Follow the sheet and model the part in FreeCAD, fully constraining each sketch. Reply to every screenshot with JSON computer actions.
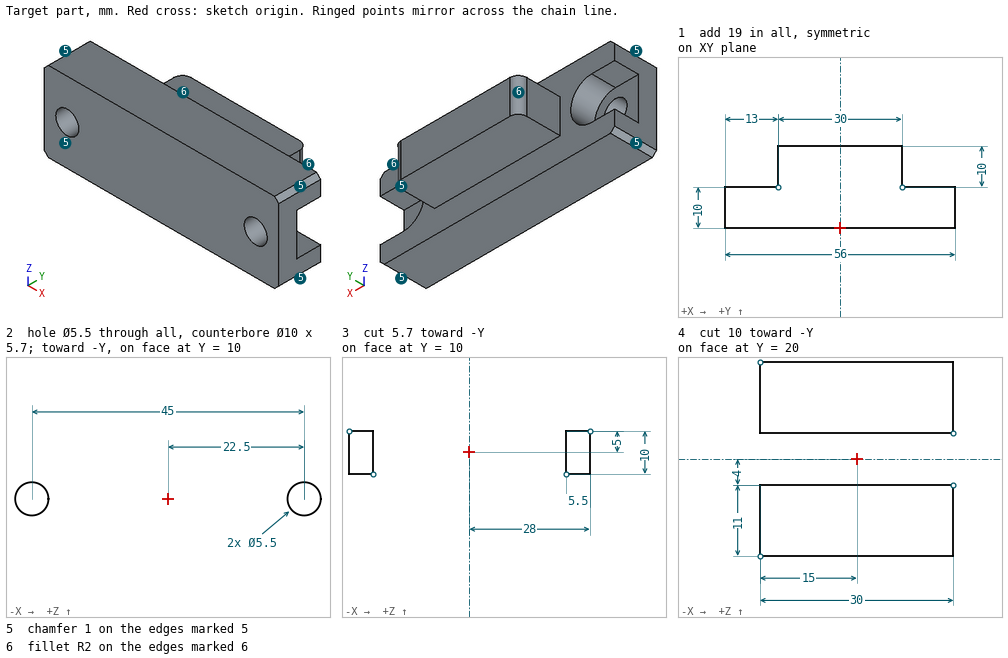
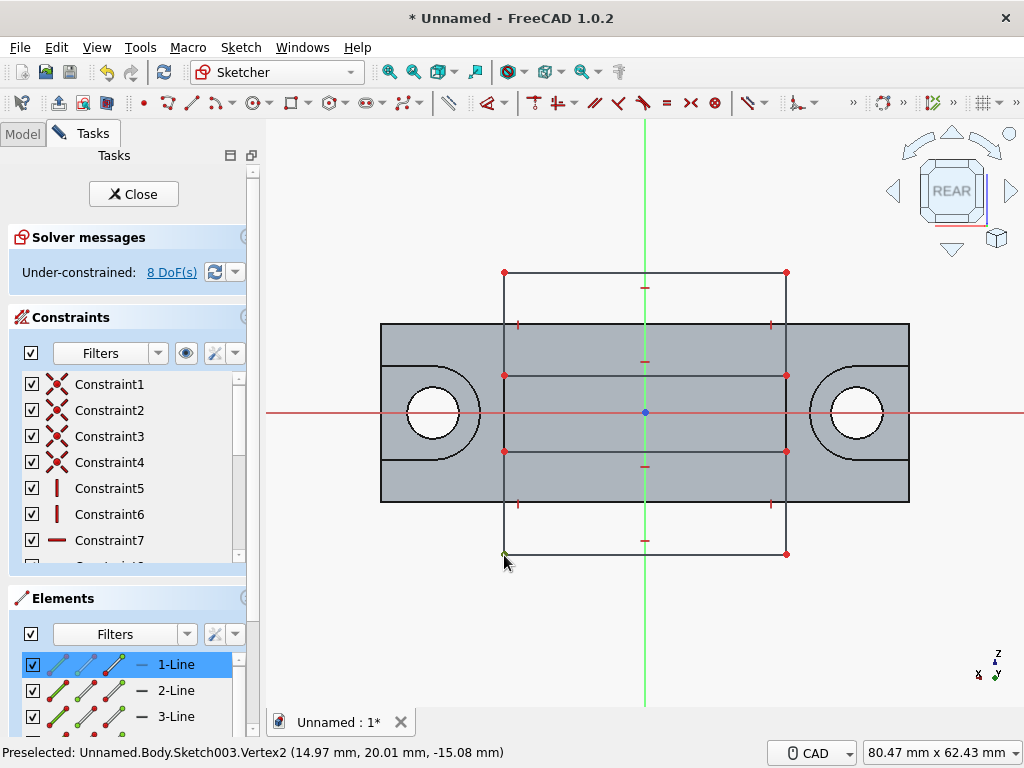
{"action": "left_click", "coordinate": [504, 273]}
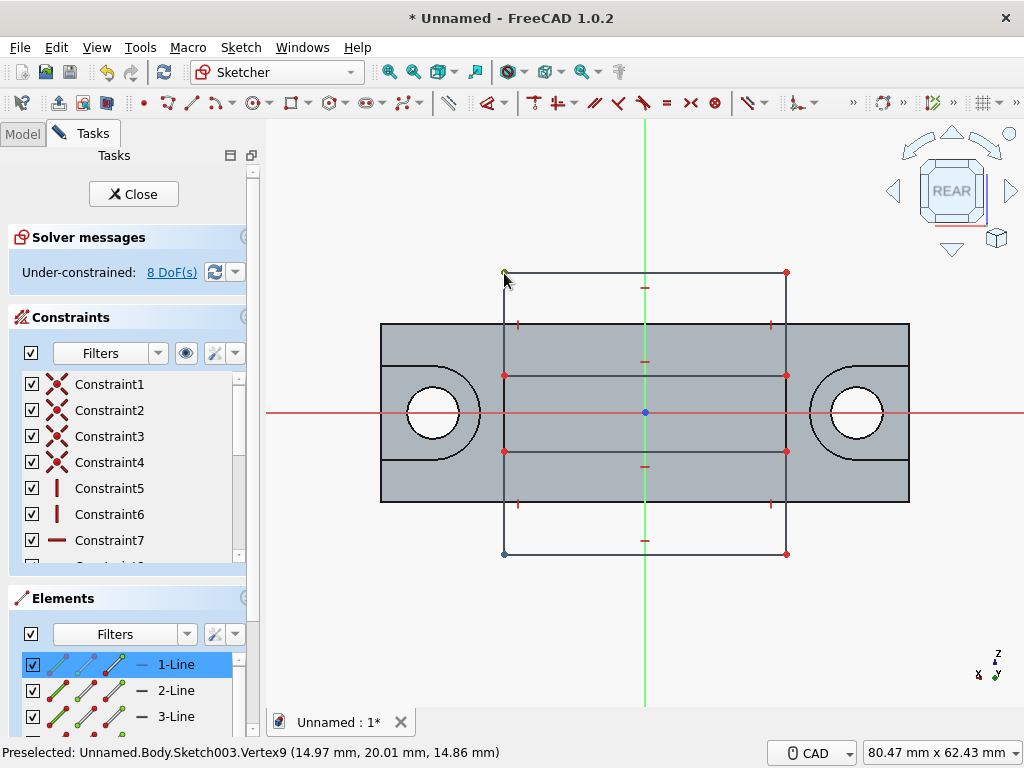
{"action": "left_click", "coordinate": [334, 413]}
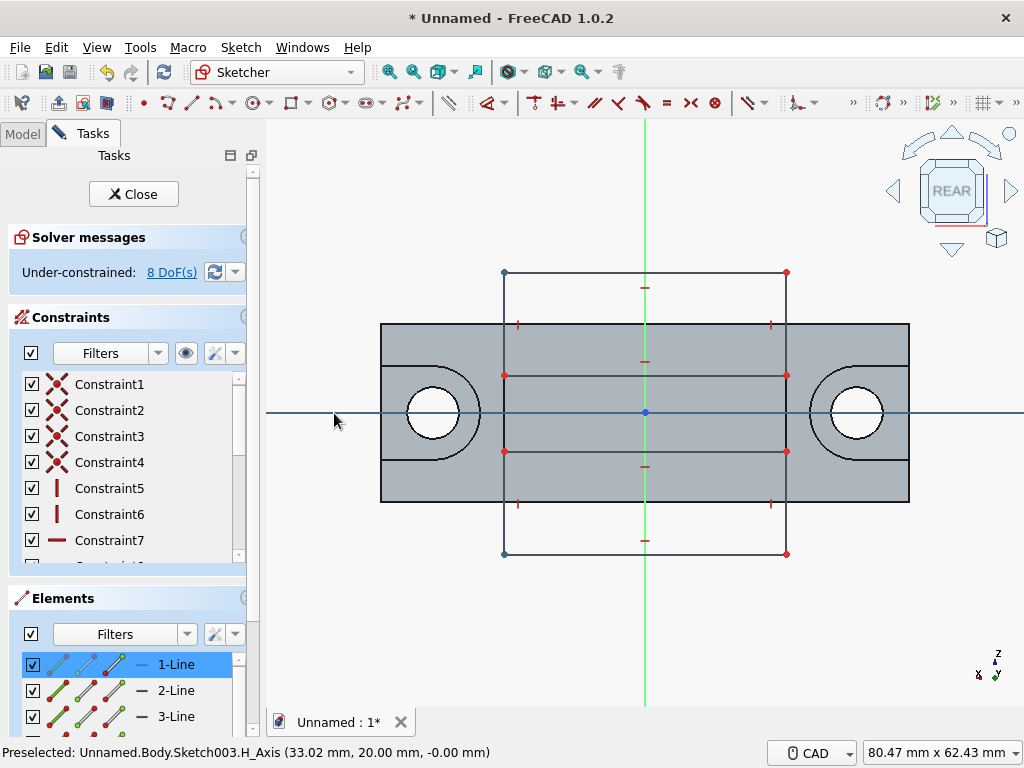
{"action": "key", "text": "s"}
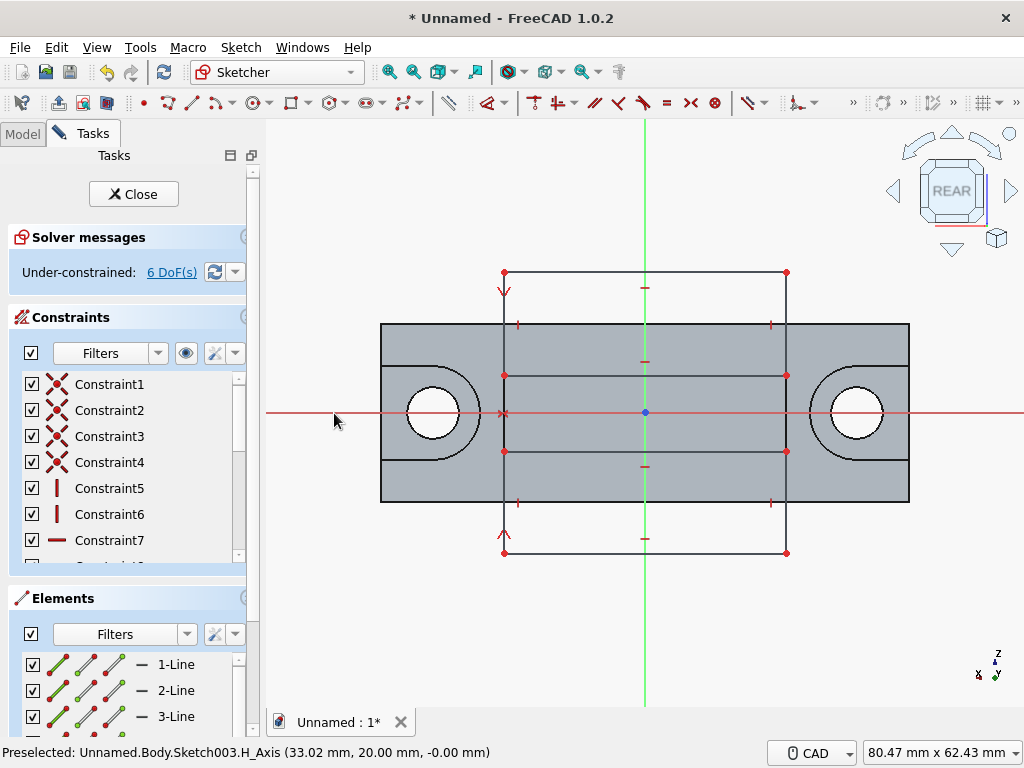
{"action": "left_click", "coordinate": [786, 452]}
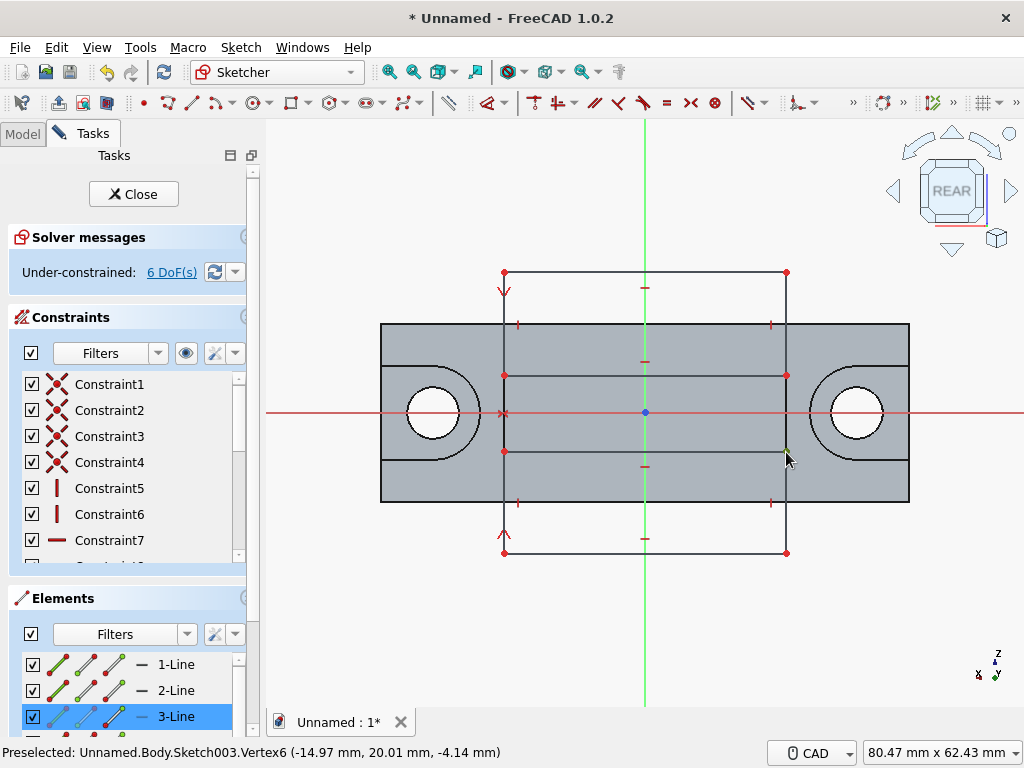
{"action": "left_click", "coordinate": [786, 376]}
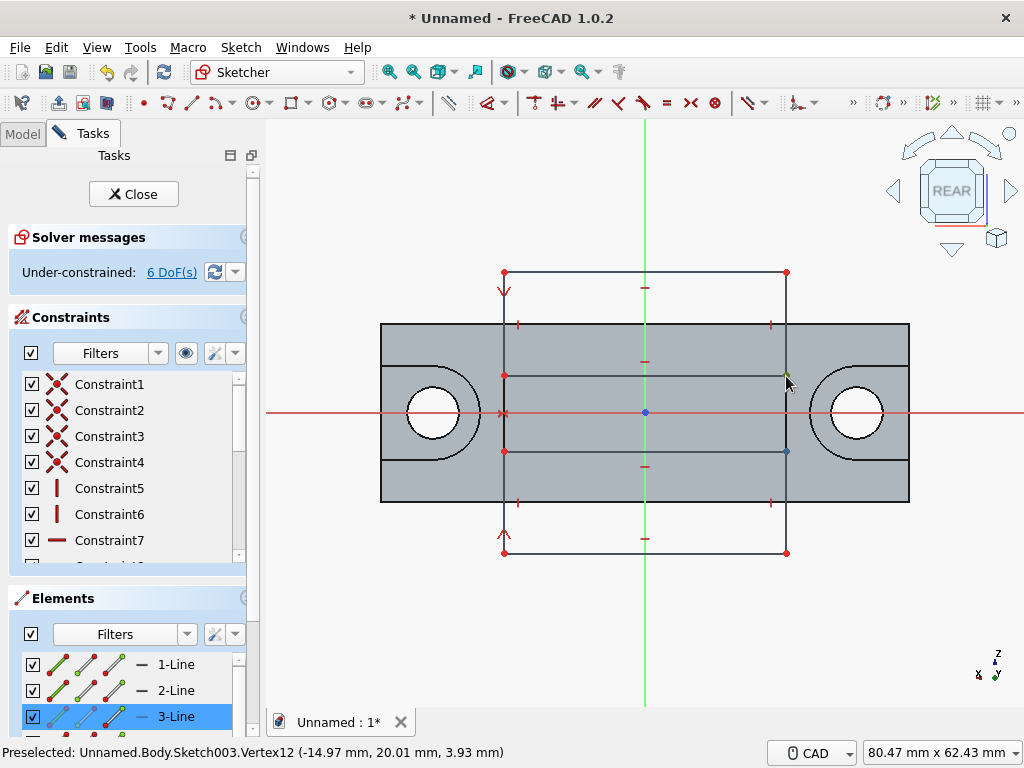
{"action": "left_click", "coordinate": [334, 413]}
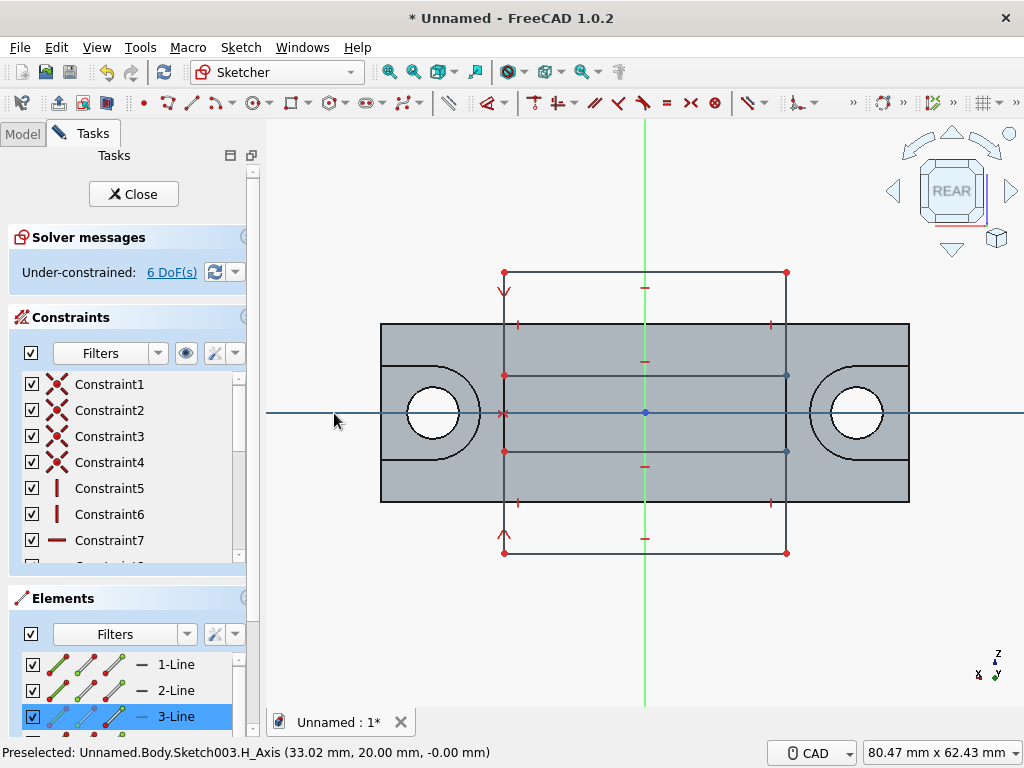
{"action": "left_click", "coordinate": [692, 104]}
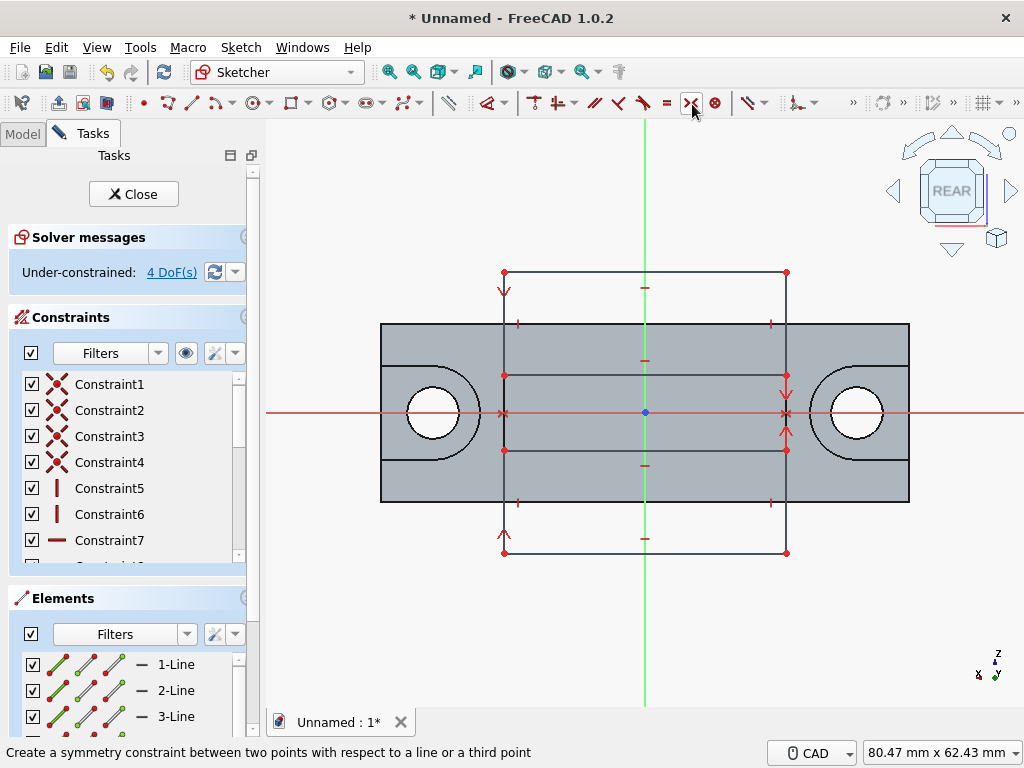
{"action": "key", "text": "d"}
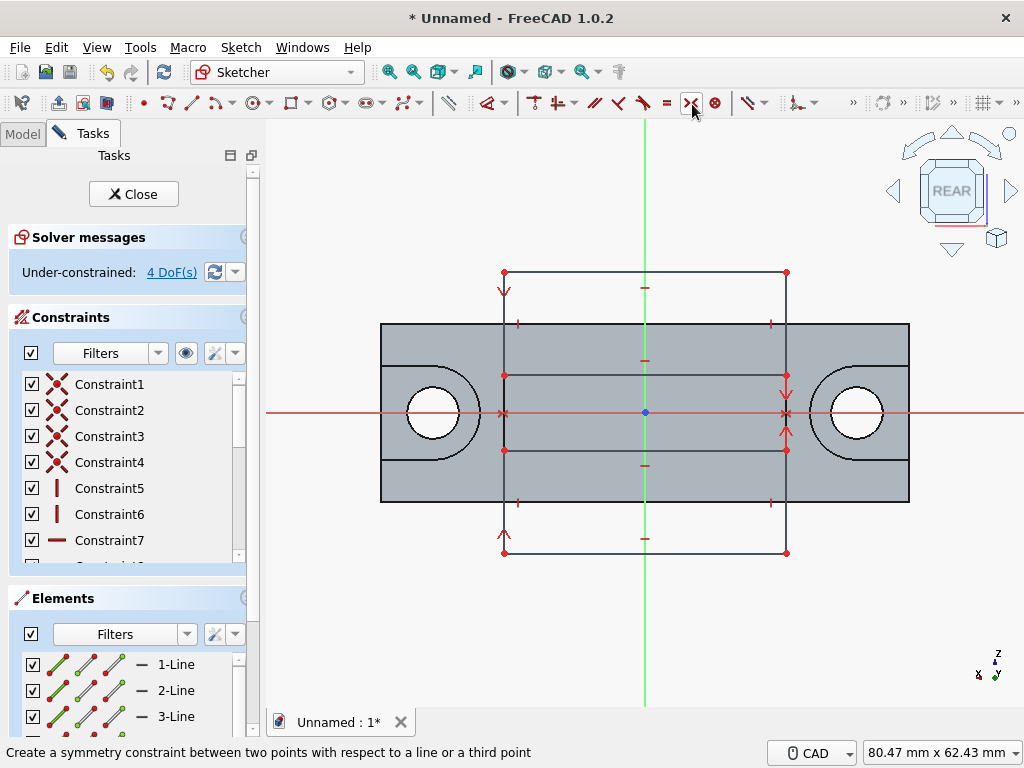
{"action": "left_click", "coordinate": [504, 482]}
{"action": "left_click", "coordinate": [470, 502]}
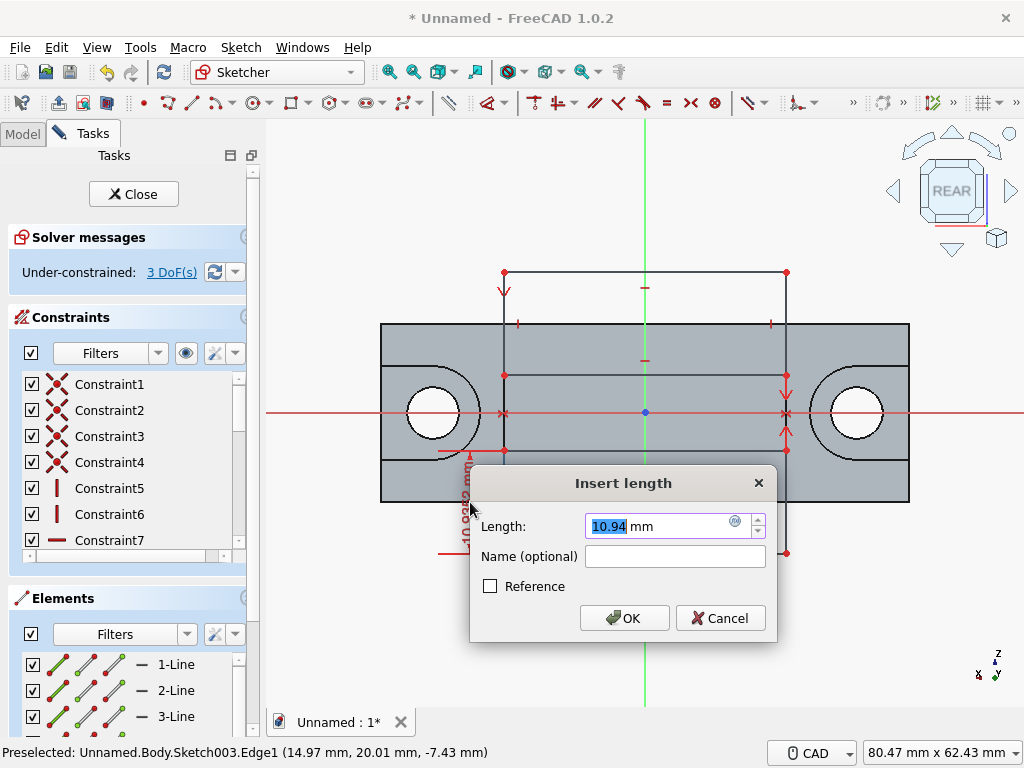
{"action": "type", "text": "11"}
{"action": "key", "text": "Return"}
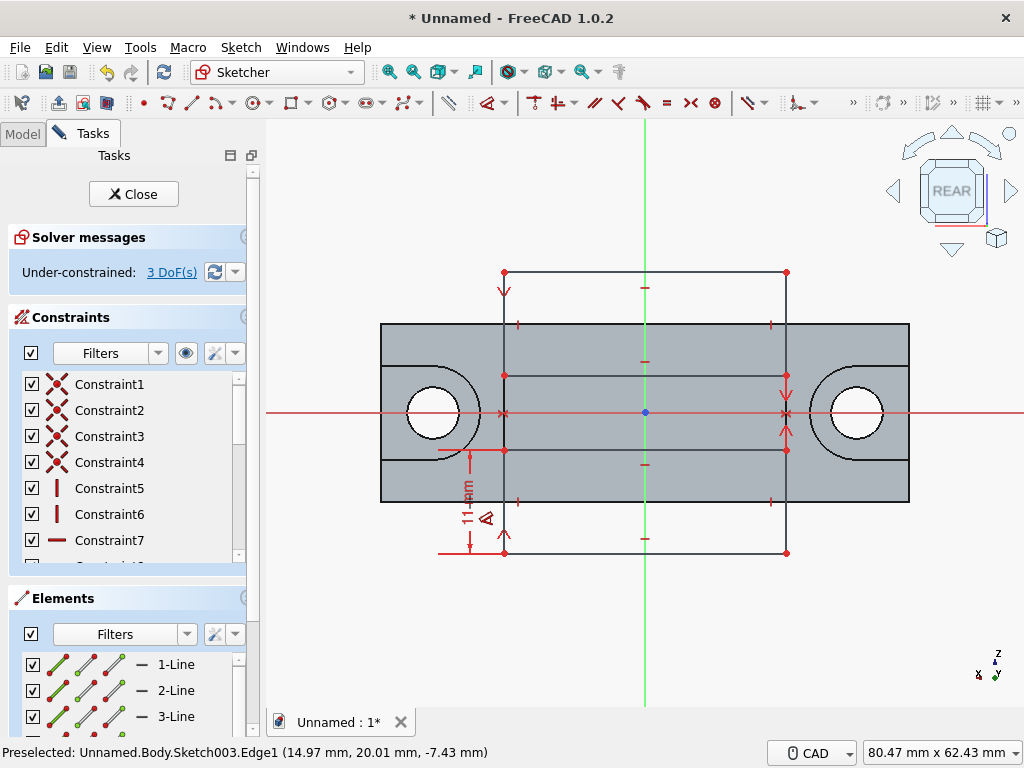
{"action": "left_click", "coordinate": [589, 554]}
{"action": "left_click", "coordinate": [580, 588]}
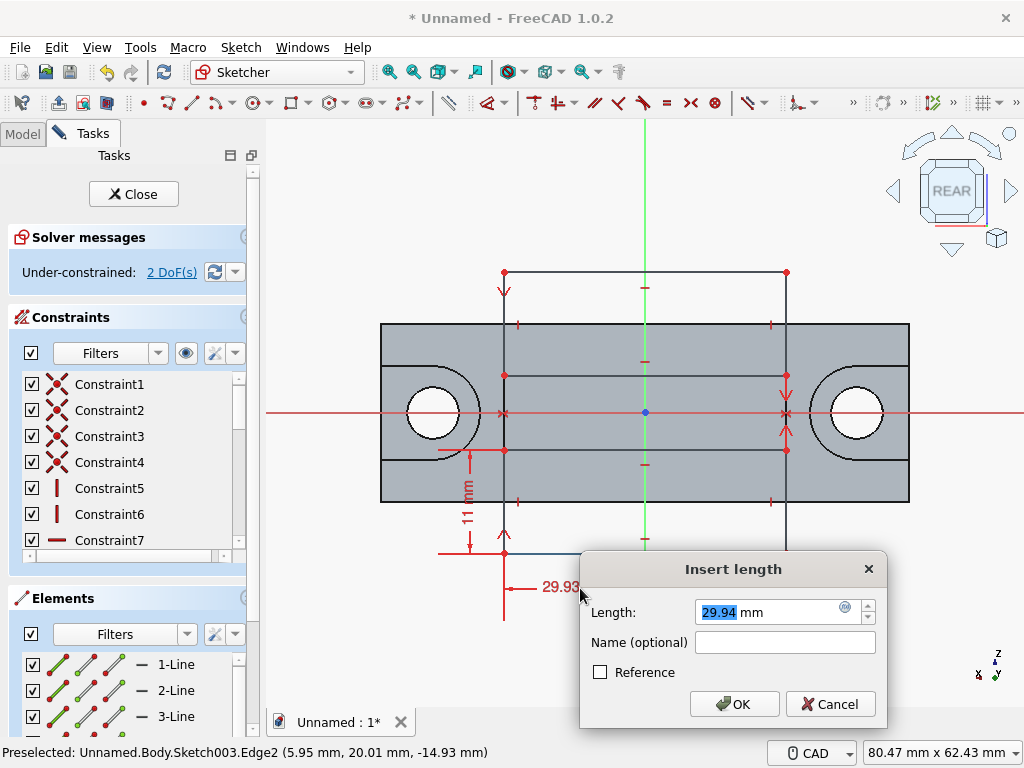
{"action": "type", "text": "30"}
{"action": "key", "text": "Return"}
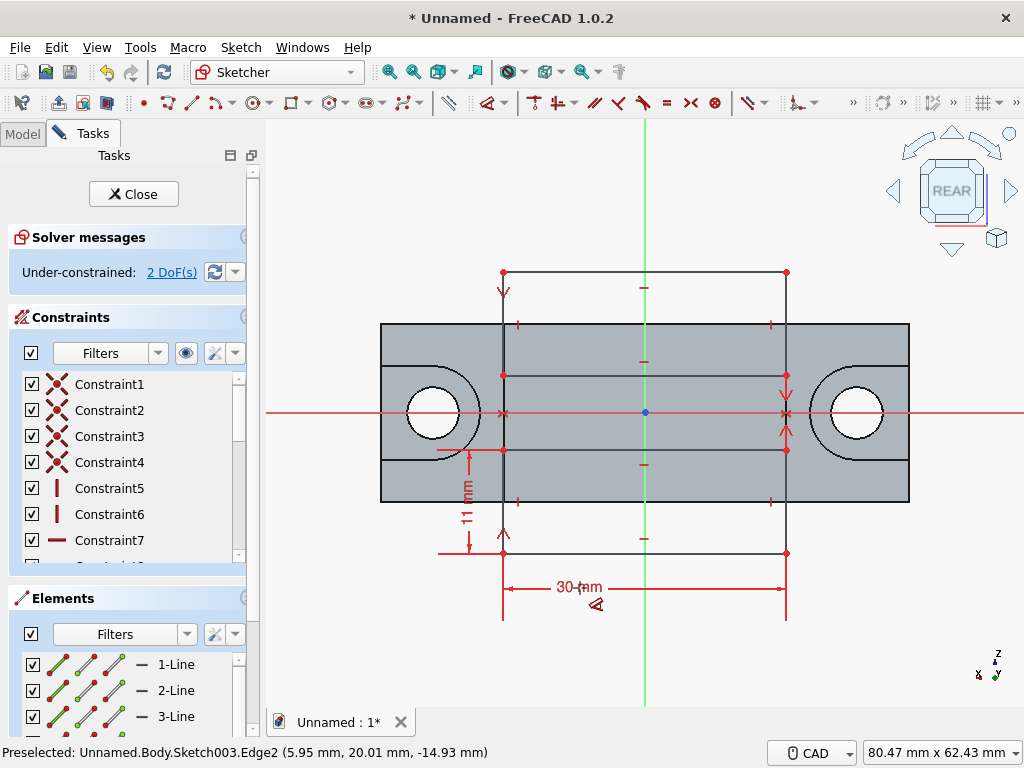
{"action": "left_click", "coordinate": [503, 450]}
{"action": "left_click", "coordinate": [469, 432]}